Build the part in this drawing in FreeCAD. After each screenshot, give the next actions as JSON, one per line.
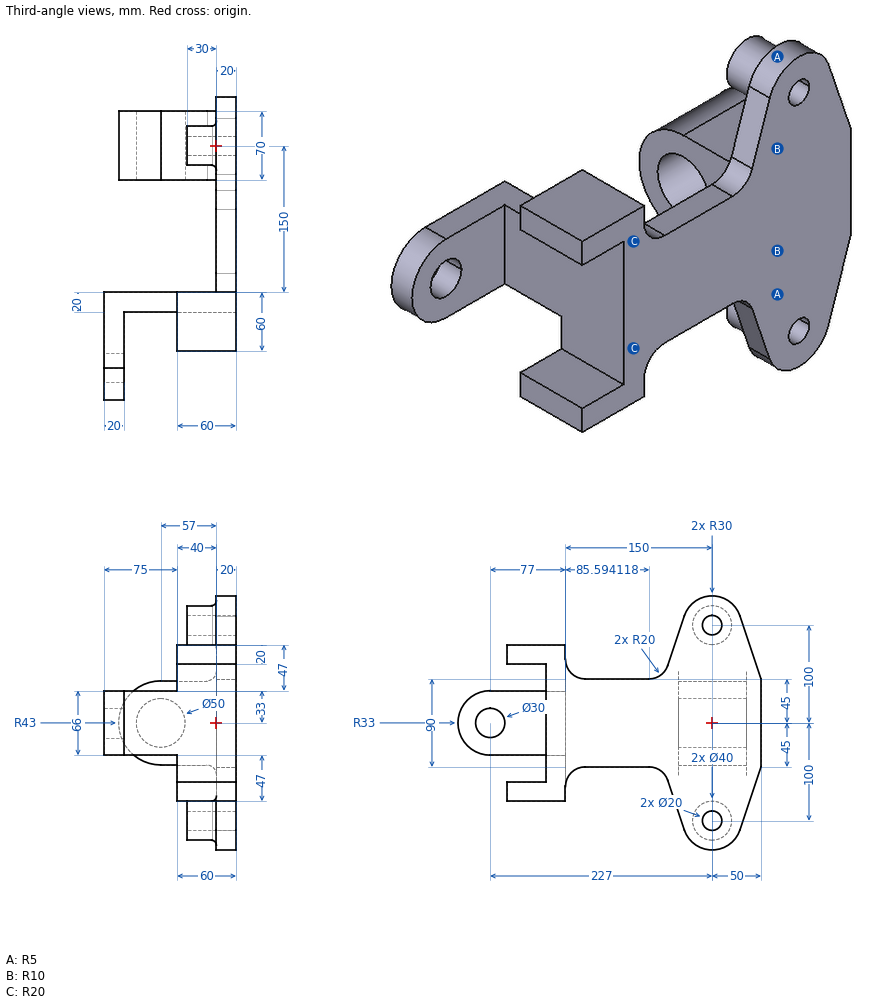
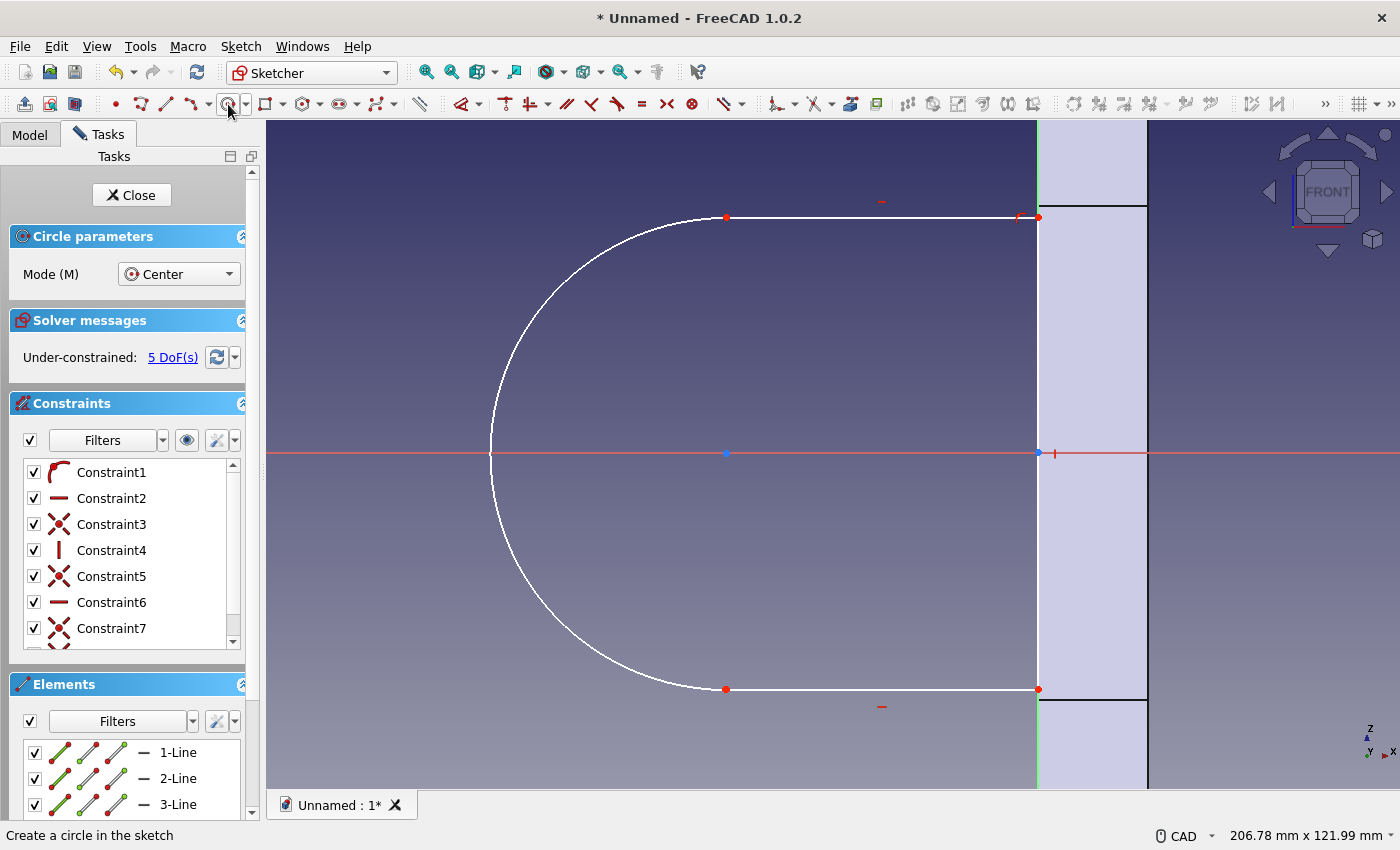
{"action": "left_click", "coordinate": [726, 453]}
{"action": "left_click", "coordinate": [823, 356]}
{"action": "key", "text": "Escape"}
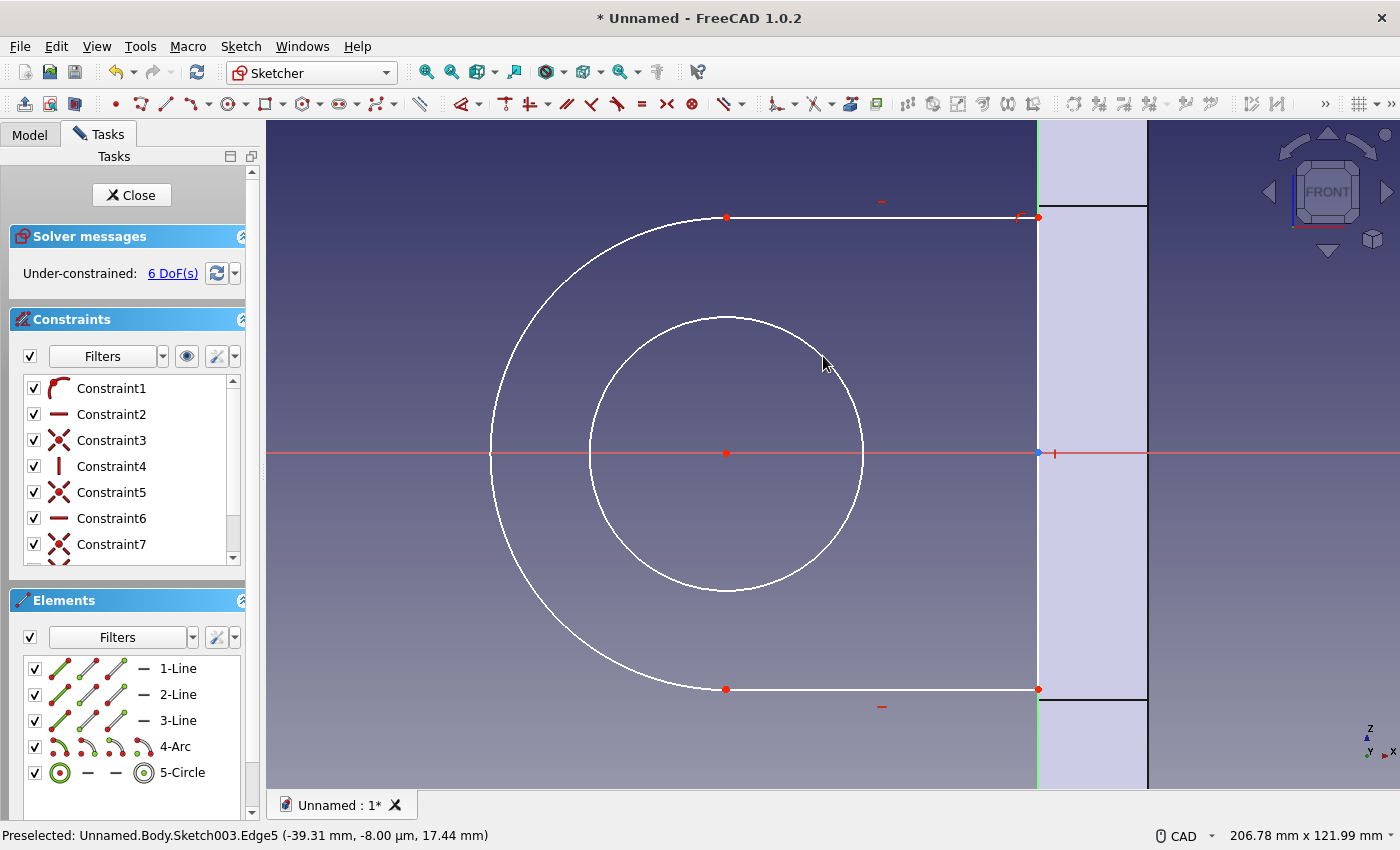
{"action": "left_click", "coordinate": [726, 454]}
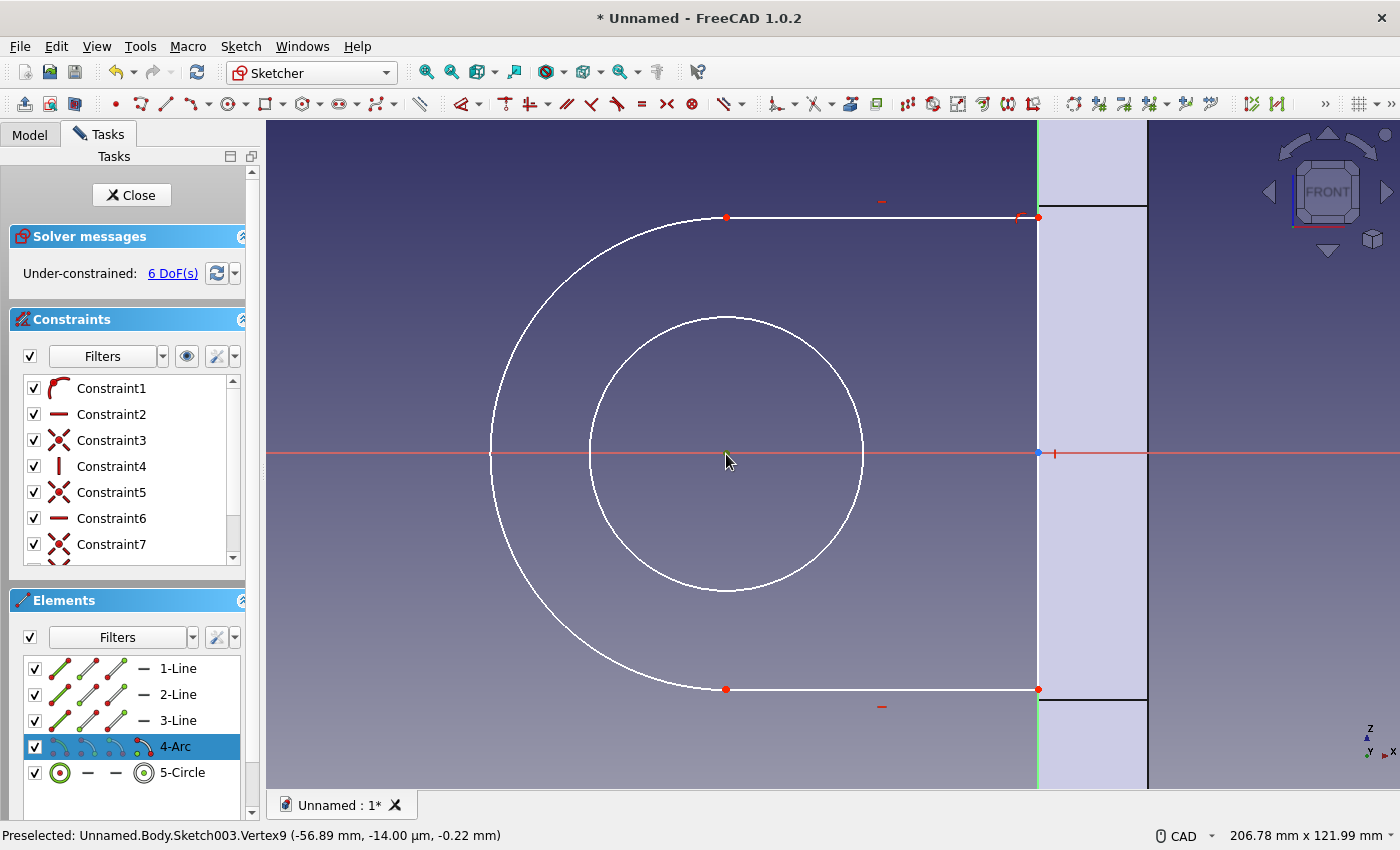
{"action": "left_click", "coordinate": [361, 453]}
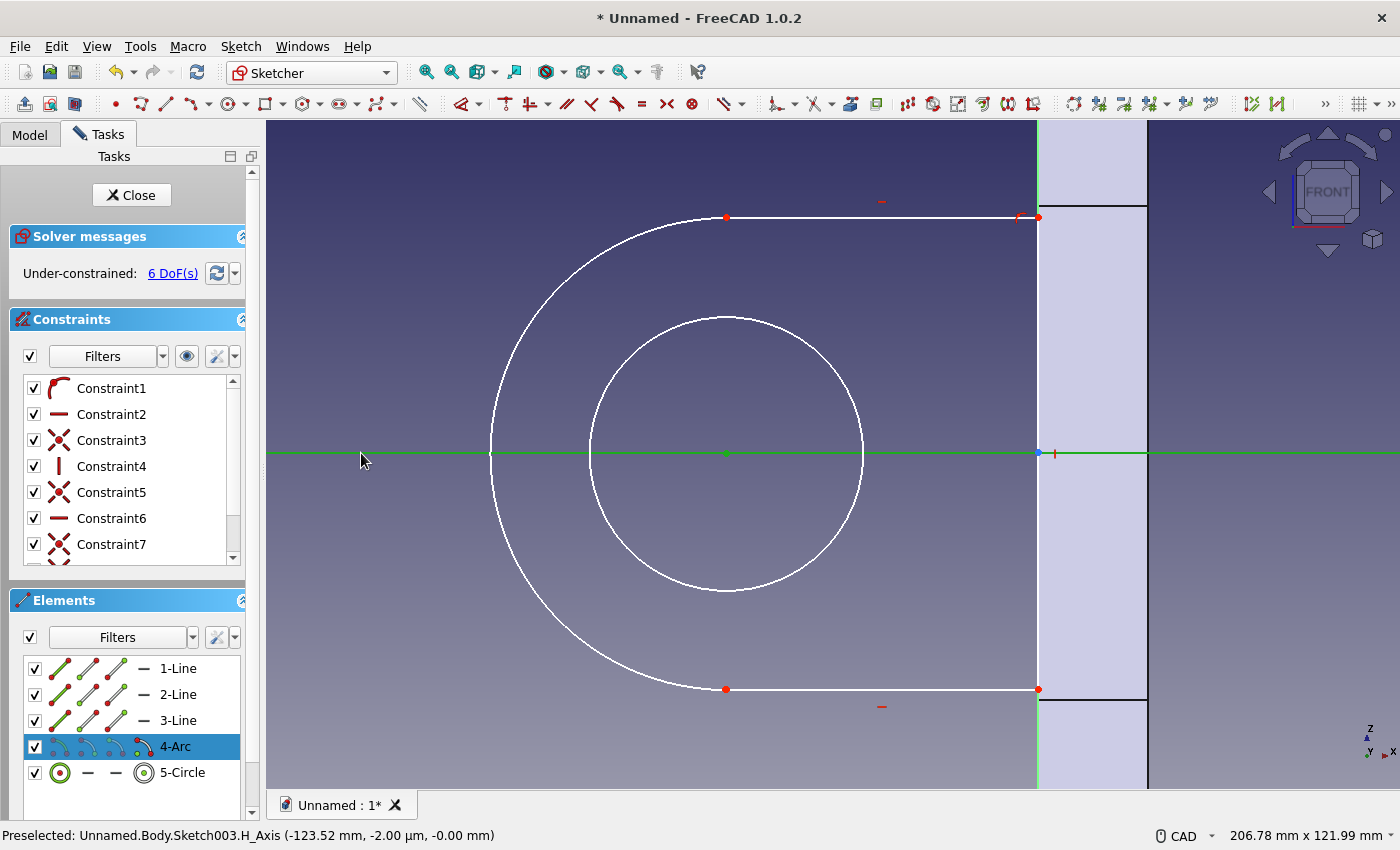
{"action": "left_click", "coordinate": [505, 104]}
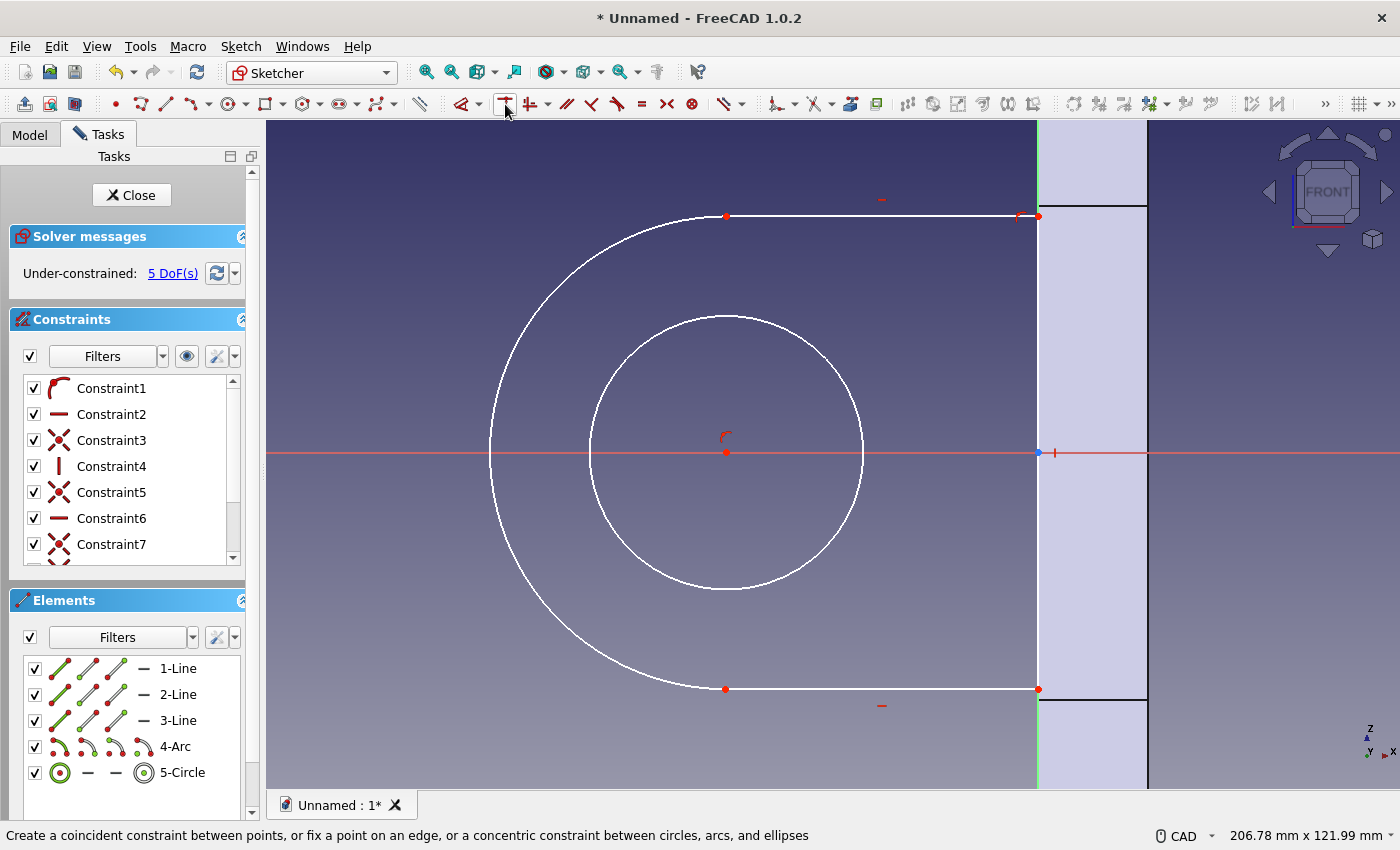
{"action": "left_click", "coordinate": [460, 104]}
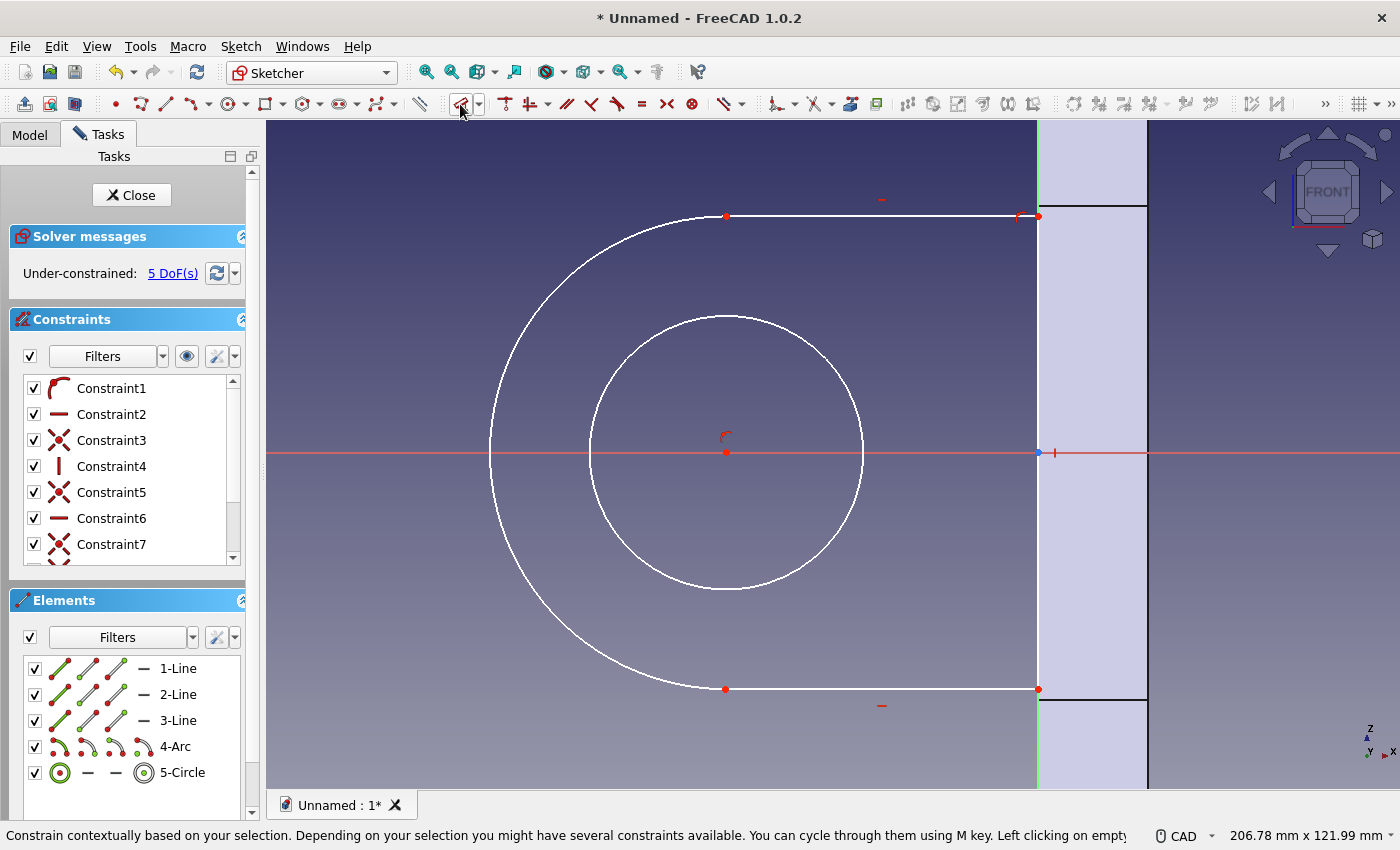
{"action": "left_click", "coordinate": [535, 314]}
{"action": "left_click", "coordinate": [509, 295]}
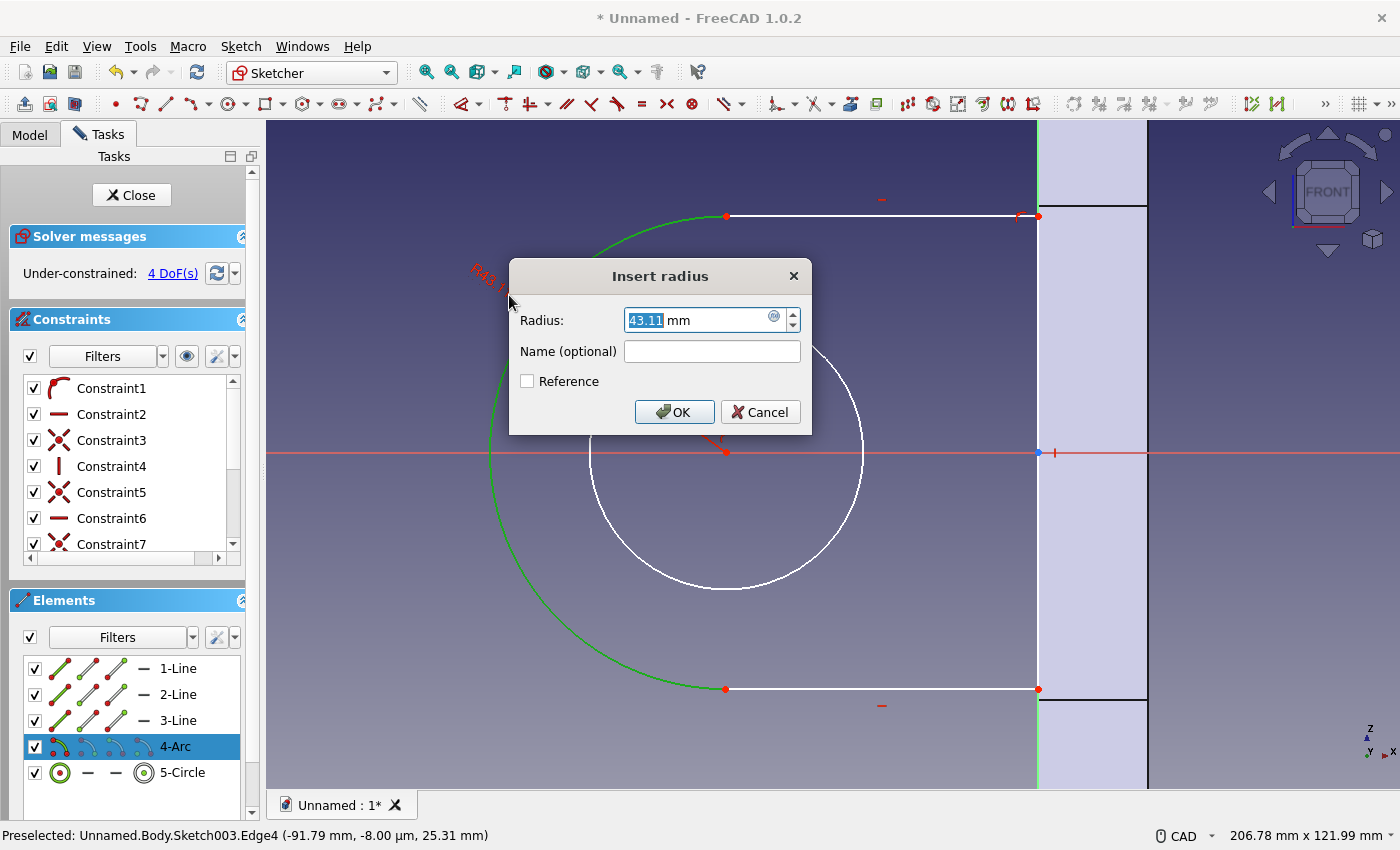
{"action": "type", "text": "43"}
{"action": "key", "text": "Return"}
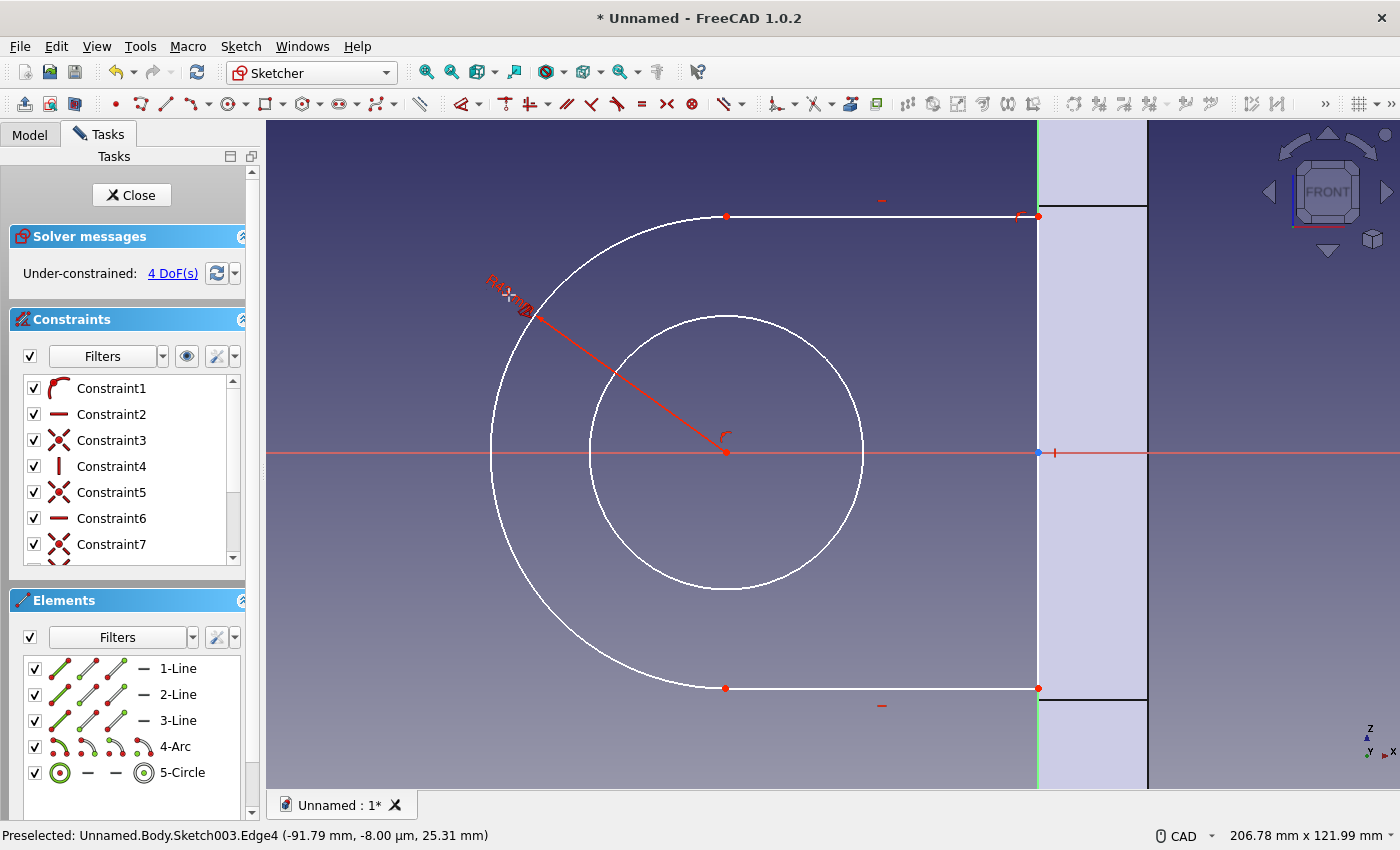
{"action": "left_click", "coordinate": [823, 356]}
{"action": "left_click", "coordinate": [846, 333]}